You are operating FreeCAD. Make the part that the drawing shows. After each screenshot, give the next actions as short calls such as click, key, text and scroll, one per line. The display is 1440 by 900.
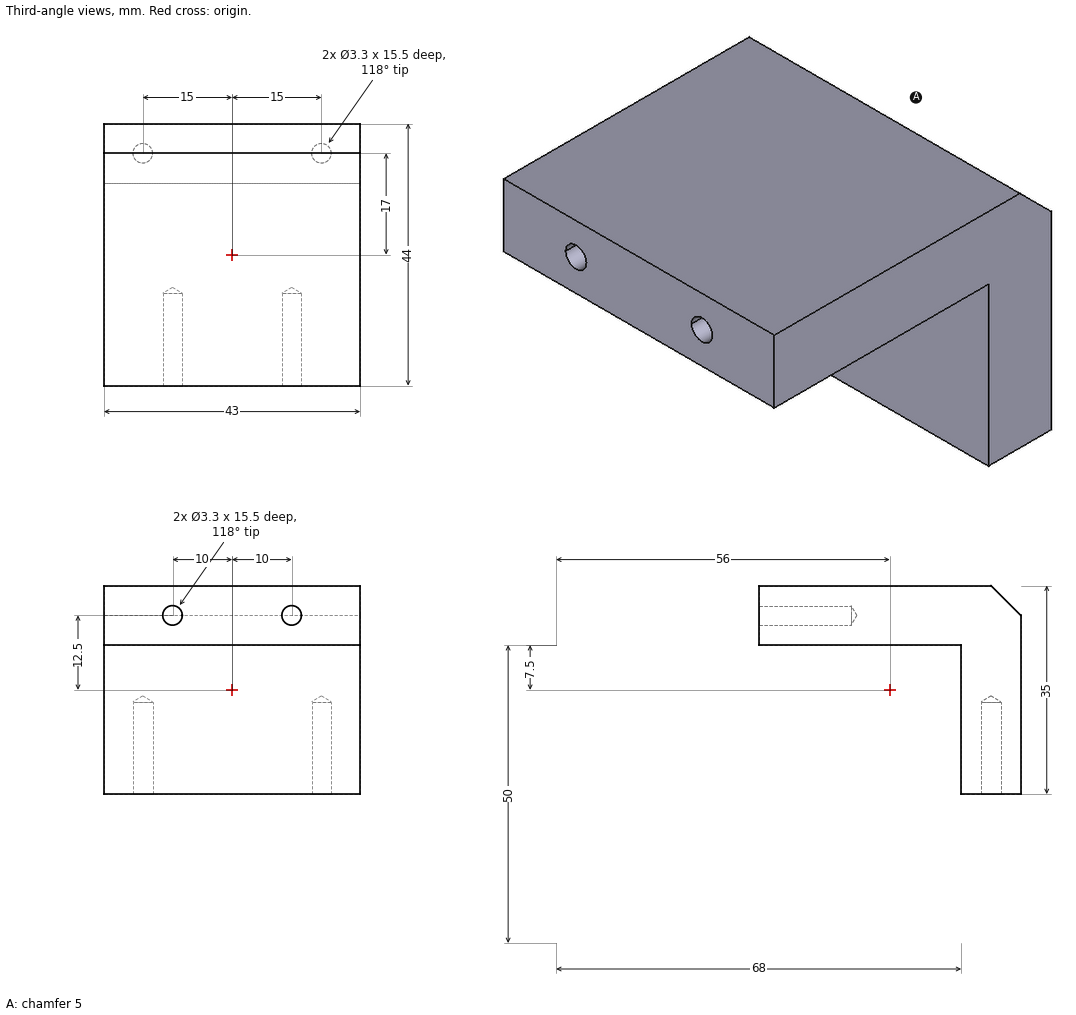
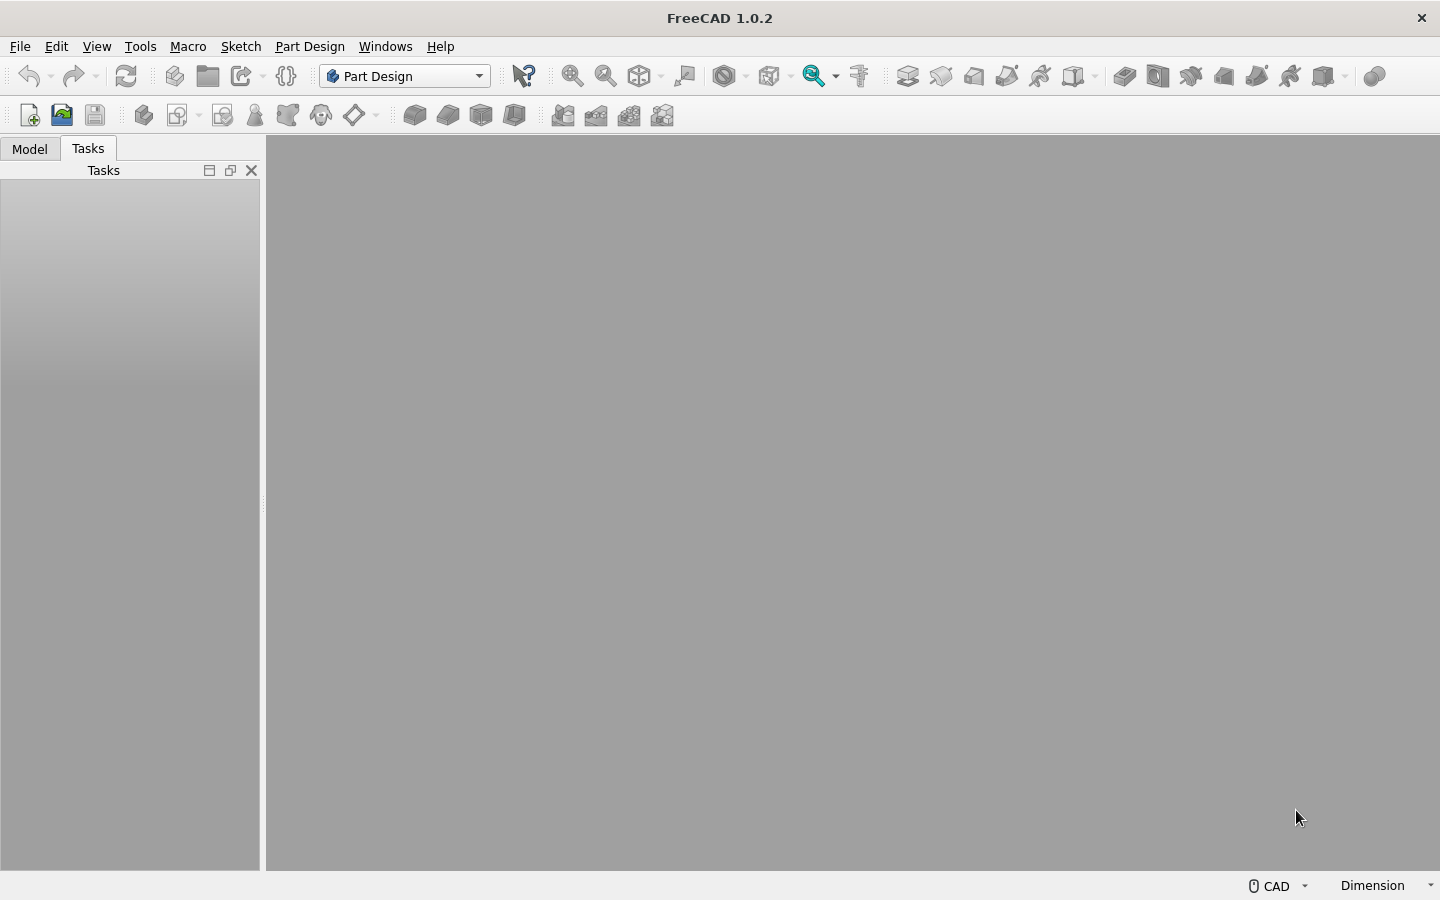
click(29, 116)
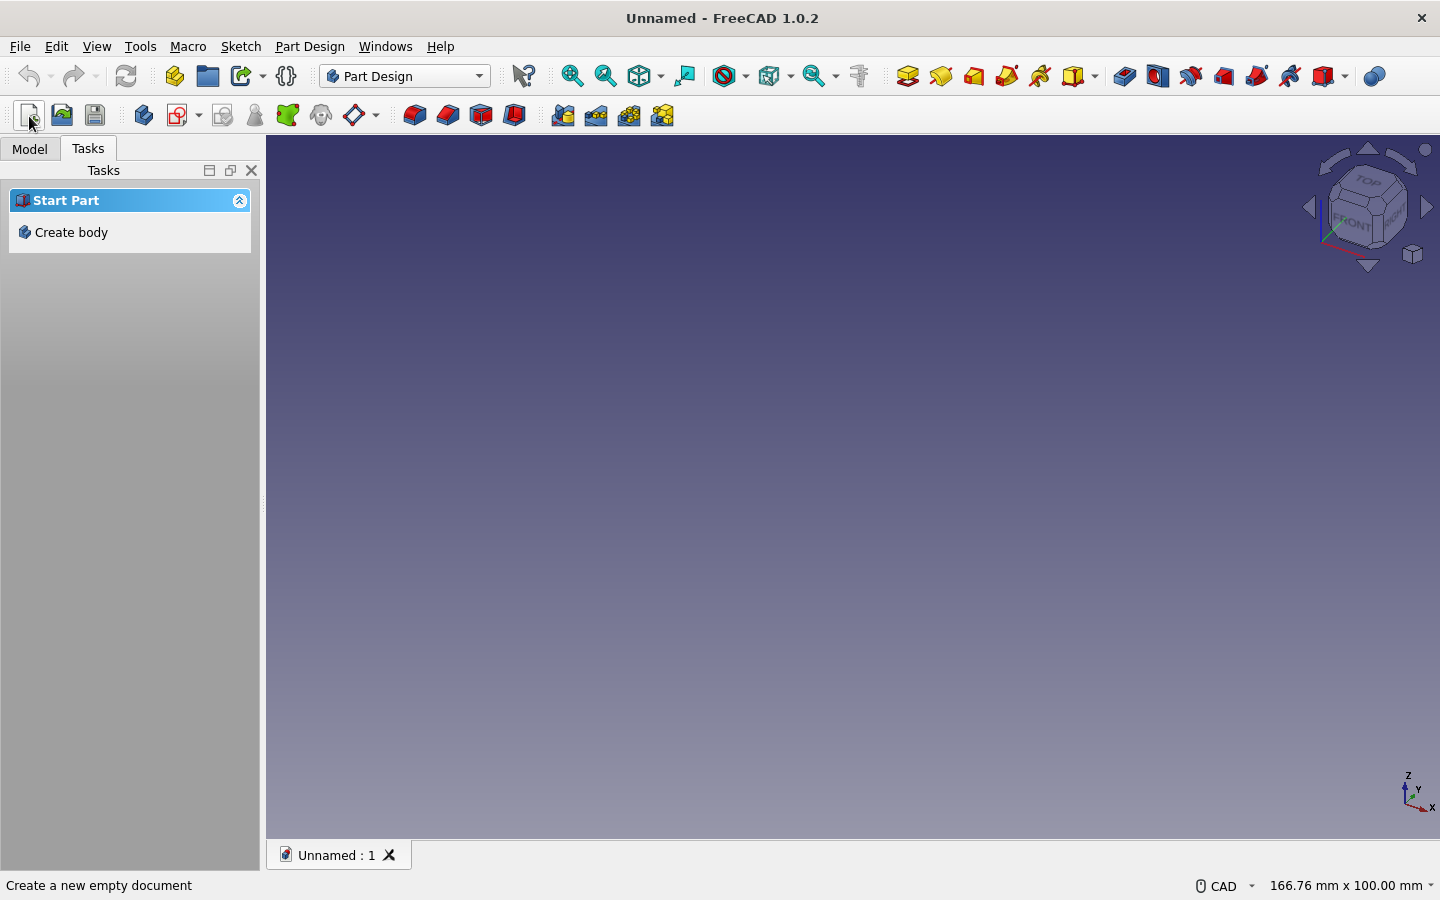
click(176, 116)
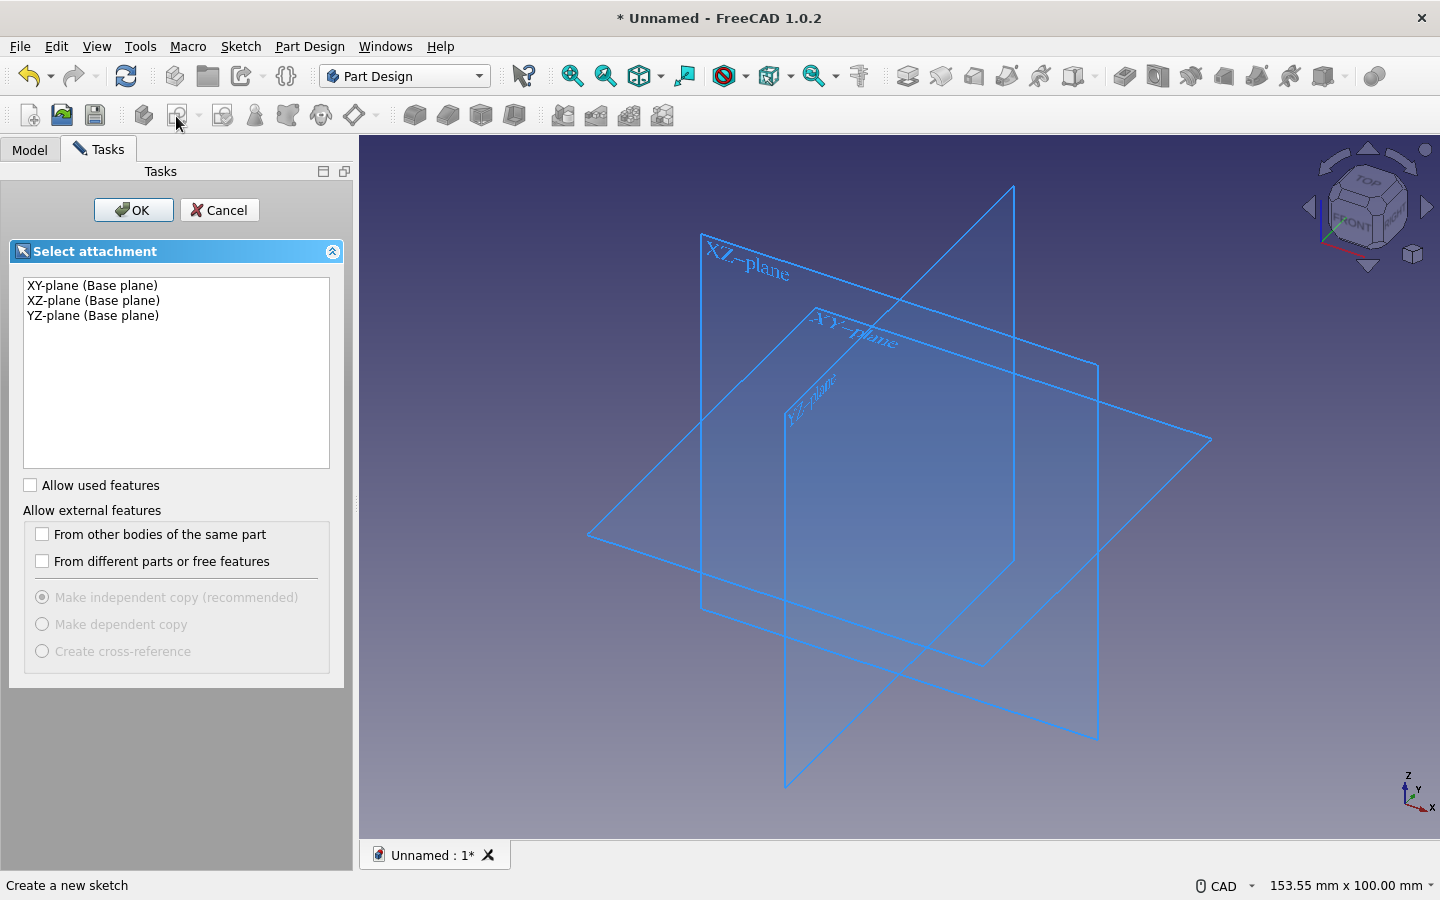
click(84, 286)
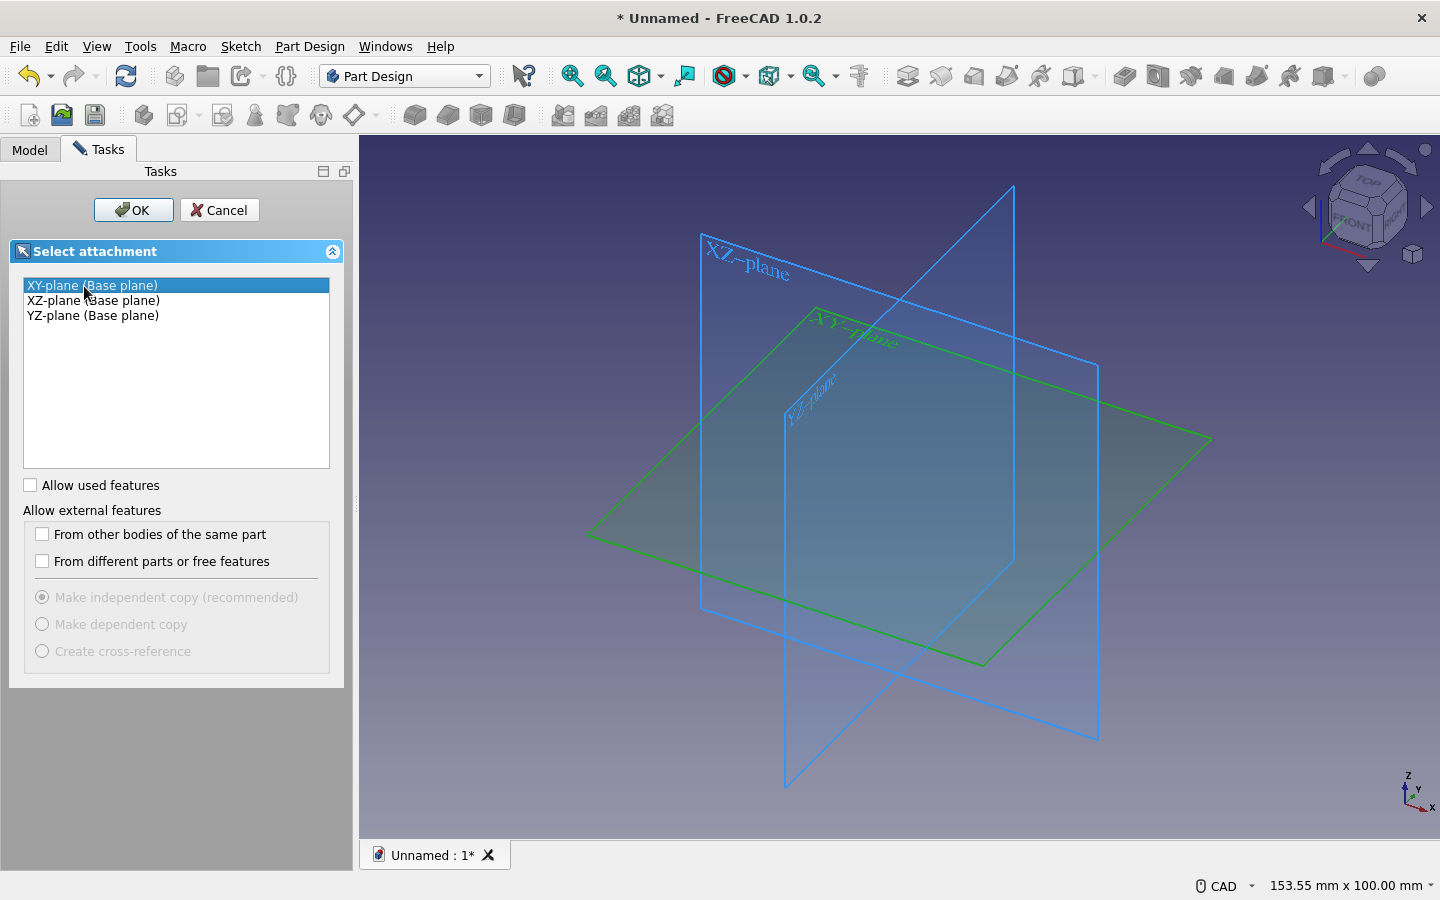
click(134, 210)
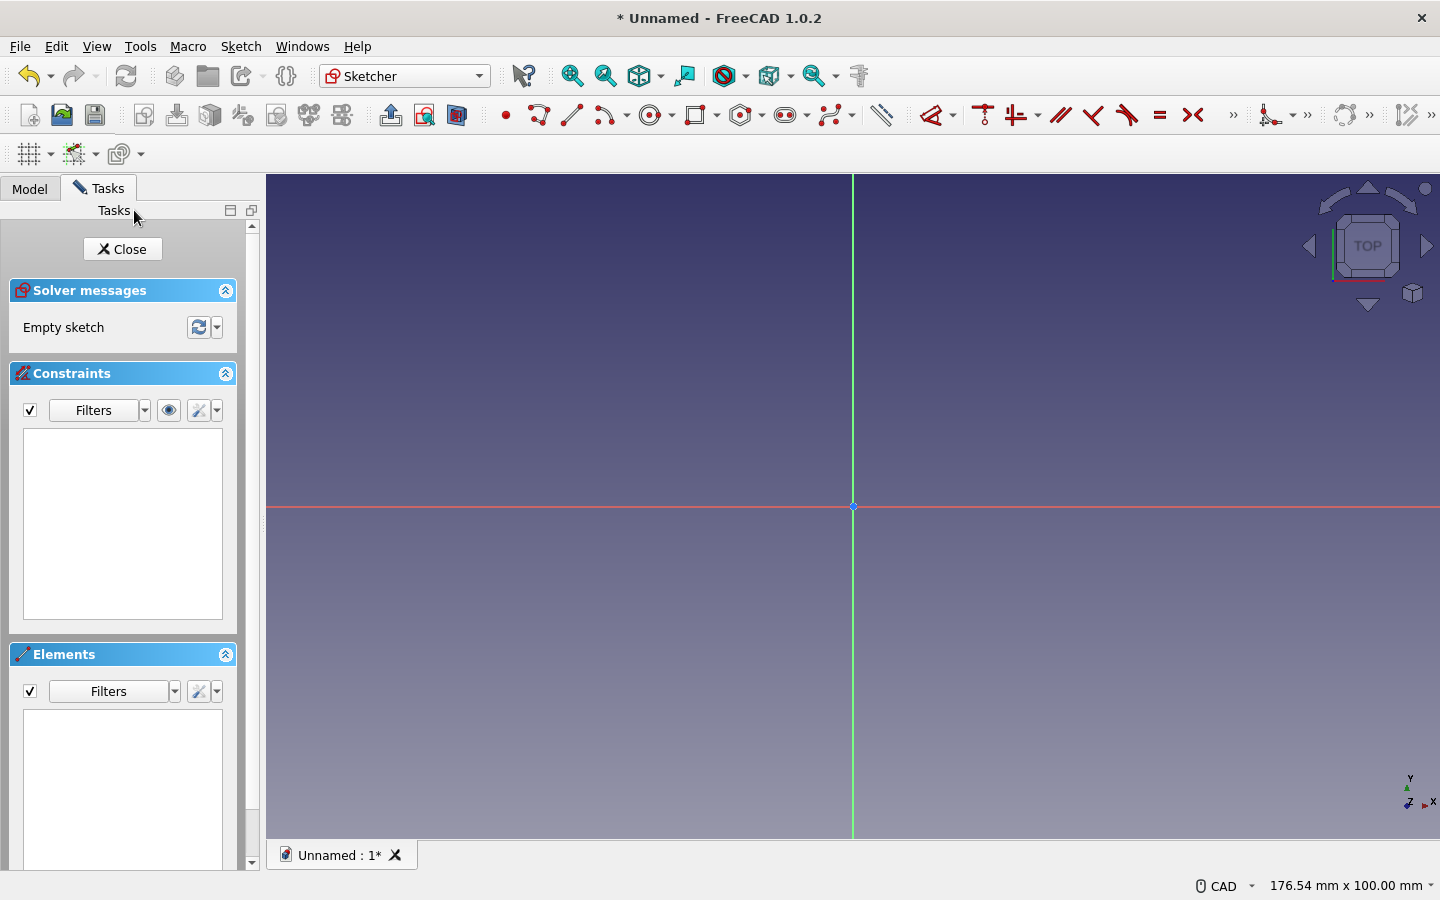
scroll(992, 506, up, 2)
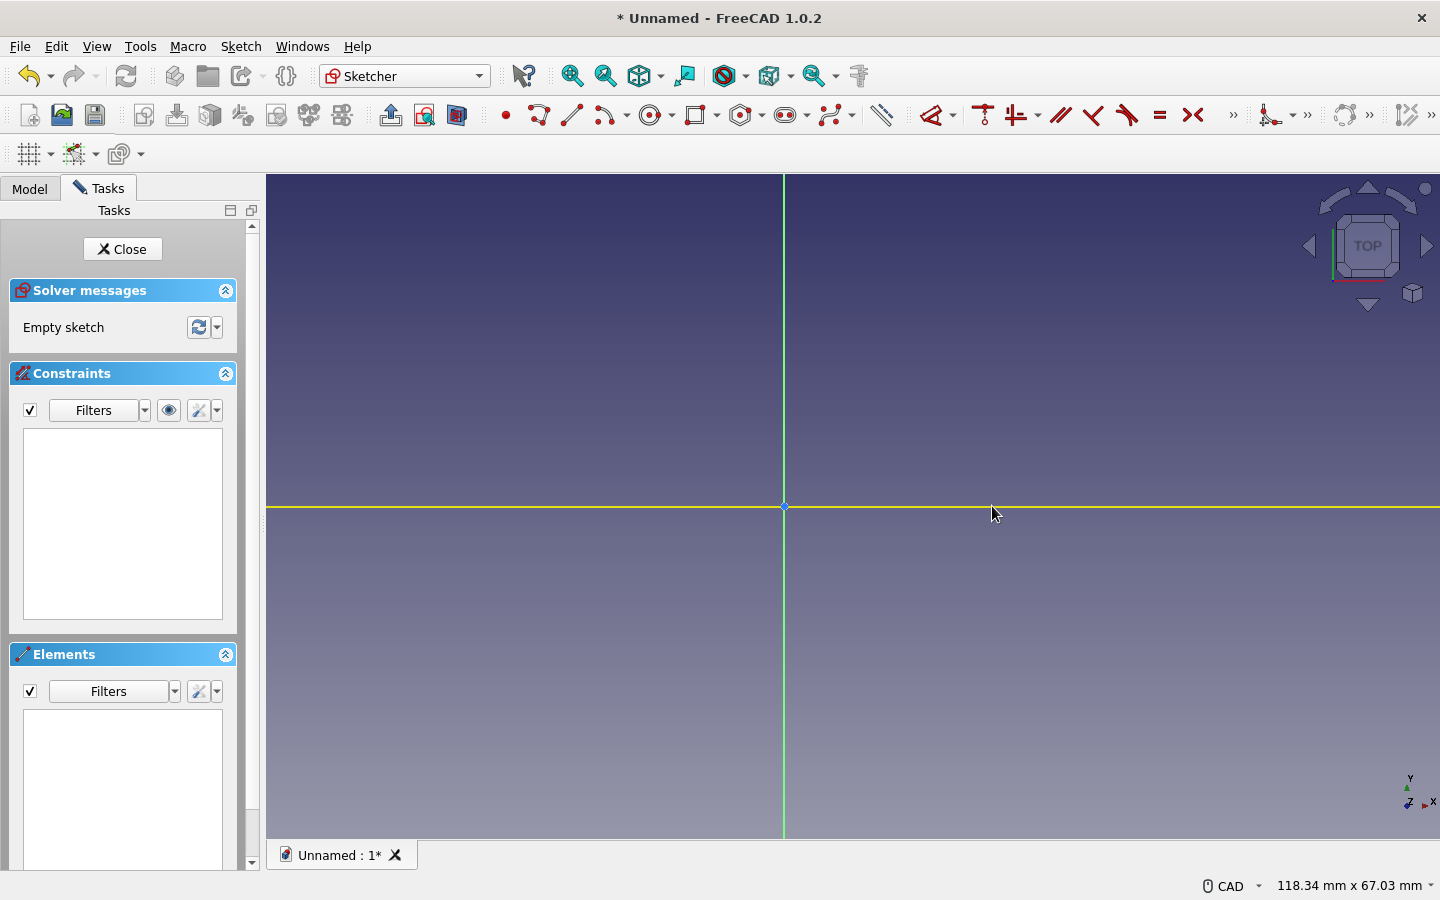
key(g)
key(v)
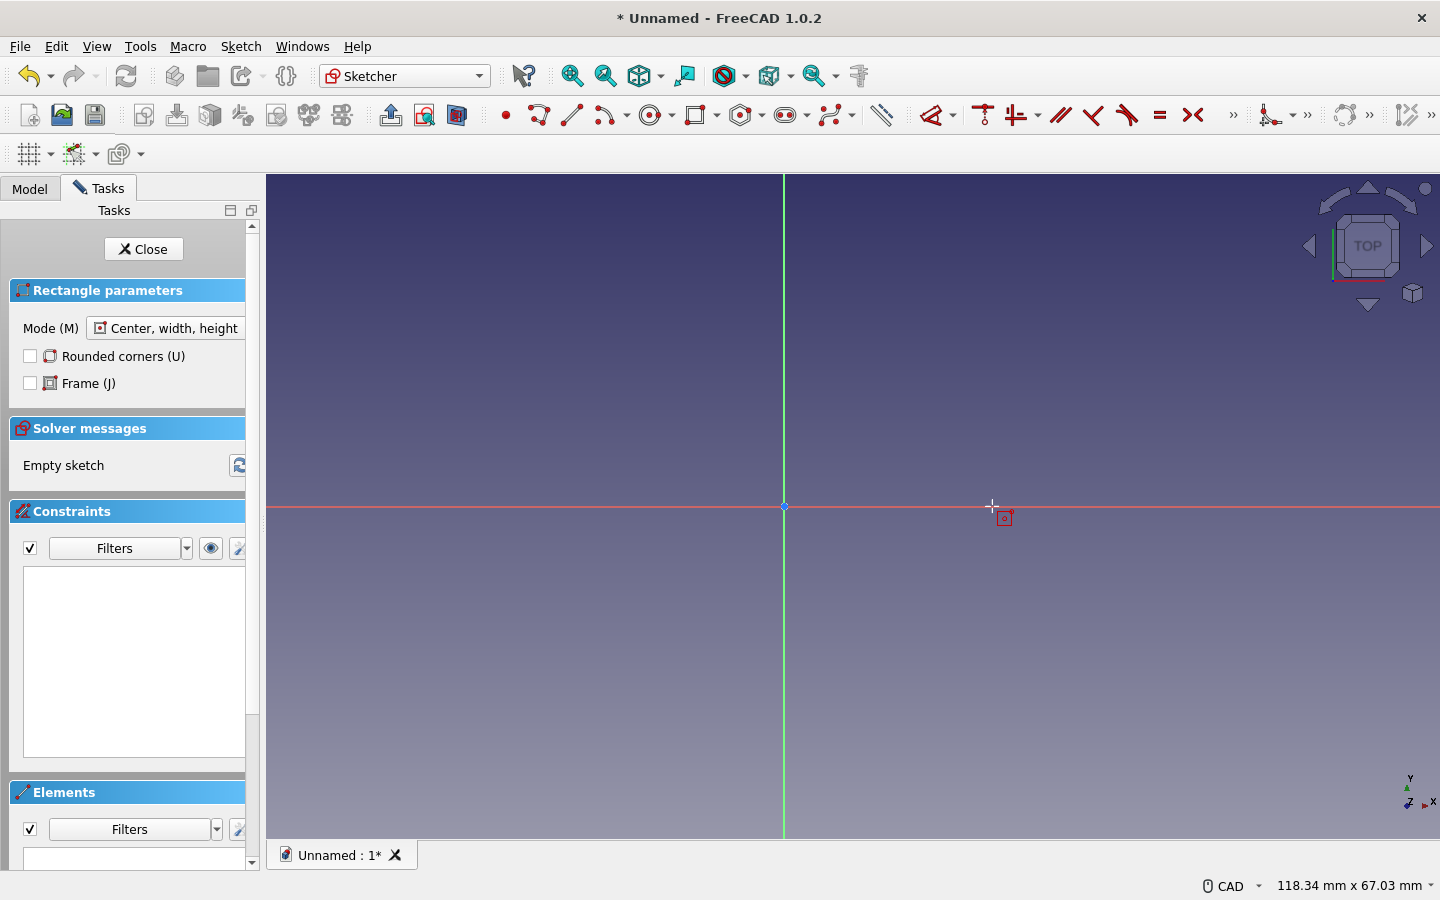
click(784, 506)
click(998, 288)
key(Escape)